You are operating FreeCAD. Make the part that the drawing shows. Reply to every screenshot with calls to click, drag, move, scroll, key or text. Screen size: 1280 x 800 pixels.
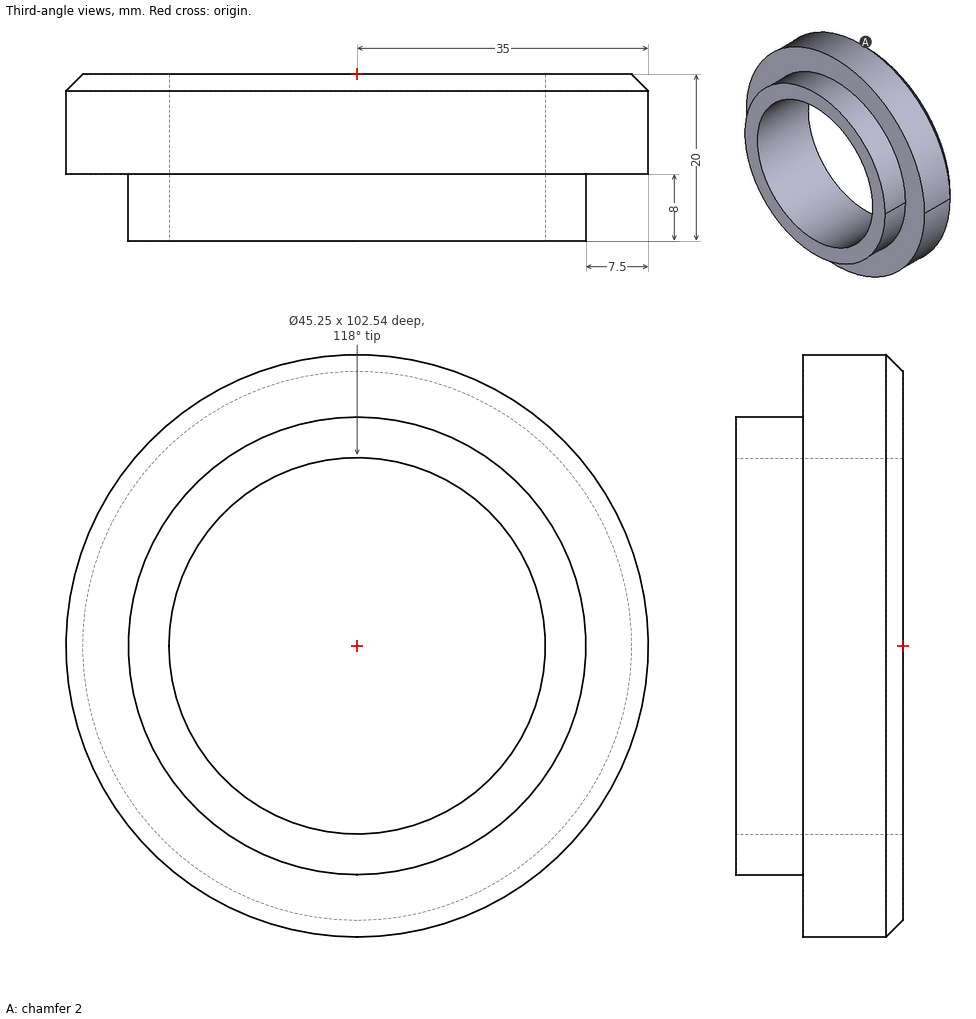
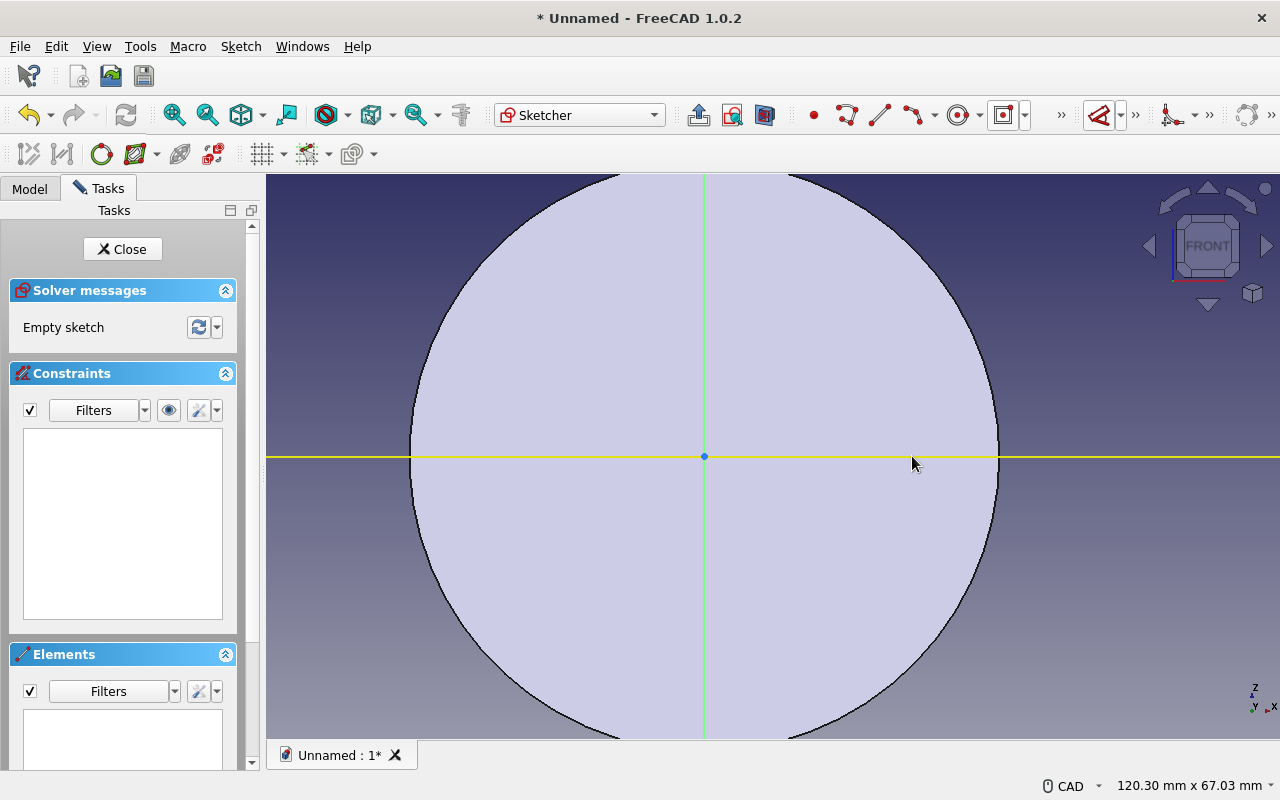
click(958, 116)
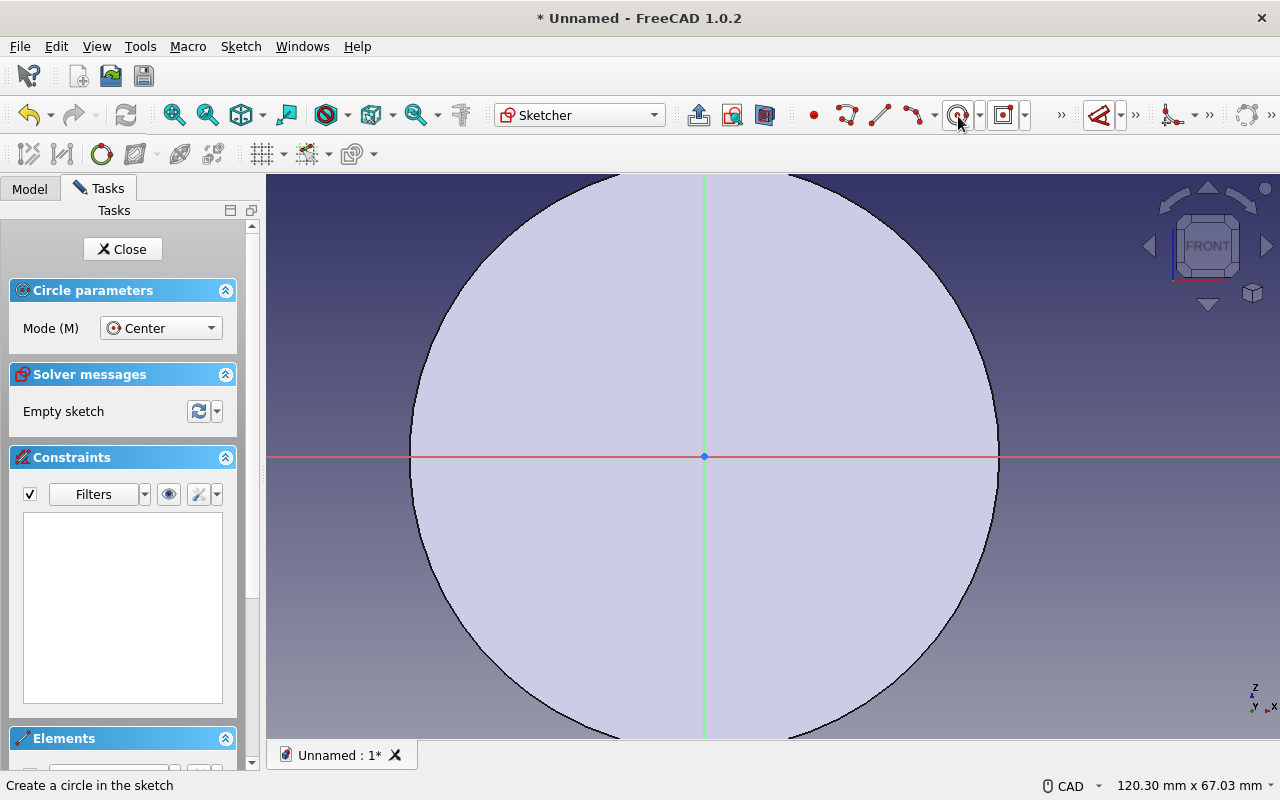
click(704, 456)
click(839, 322)
key(Escape)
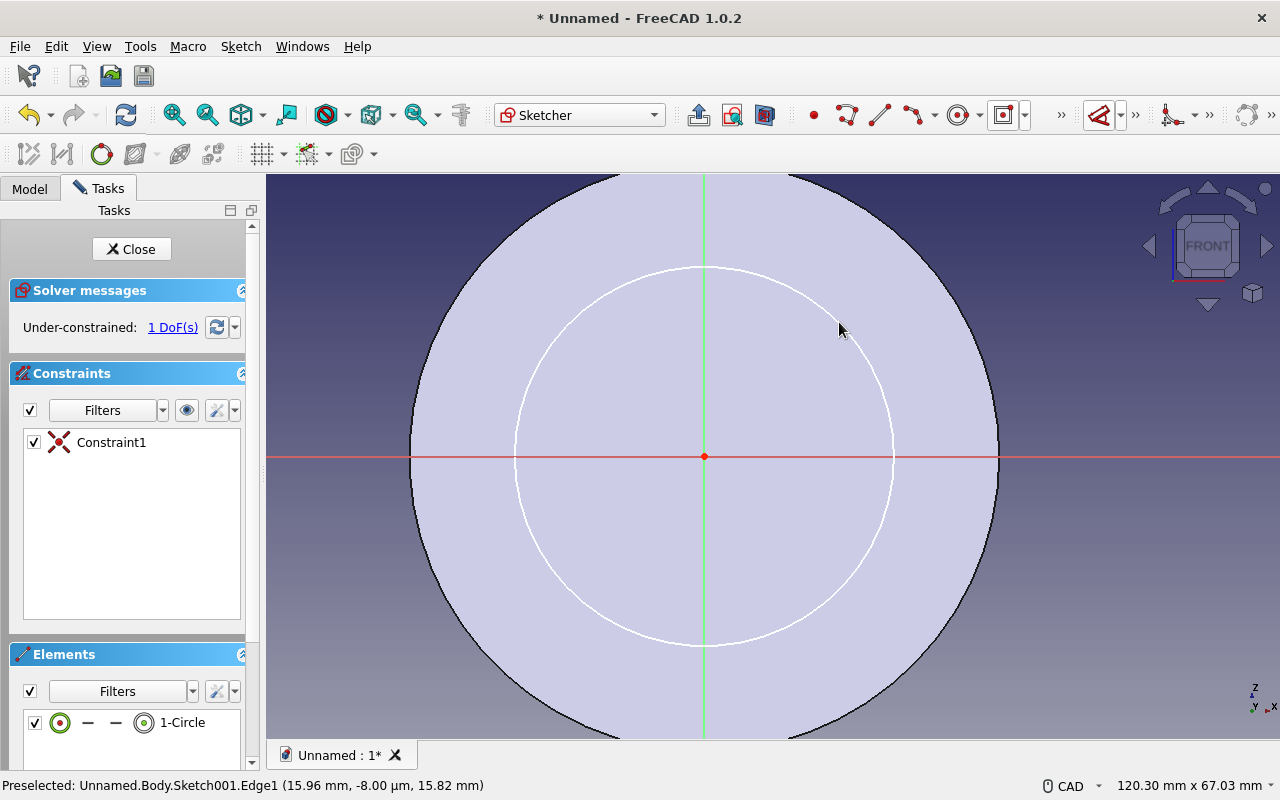
click(838, 322)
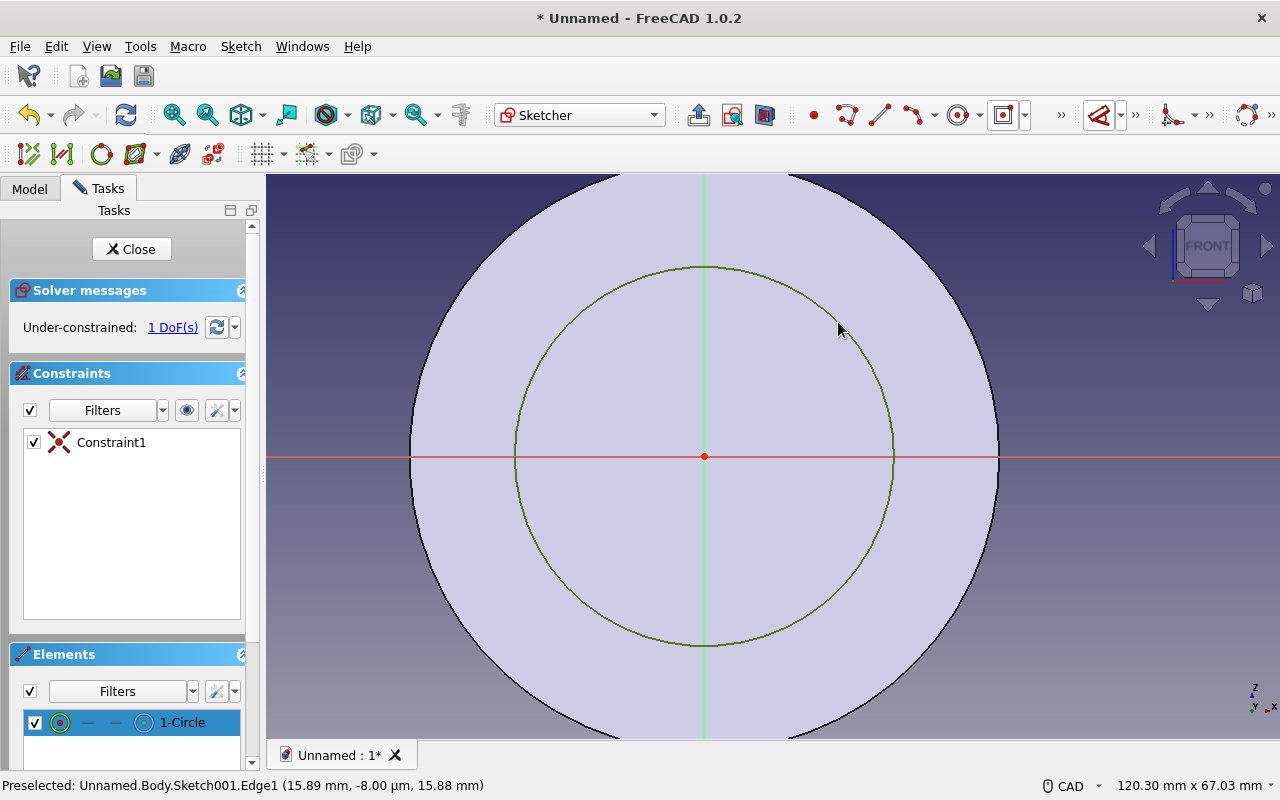
click(1120, 116)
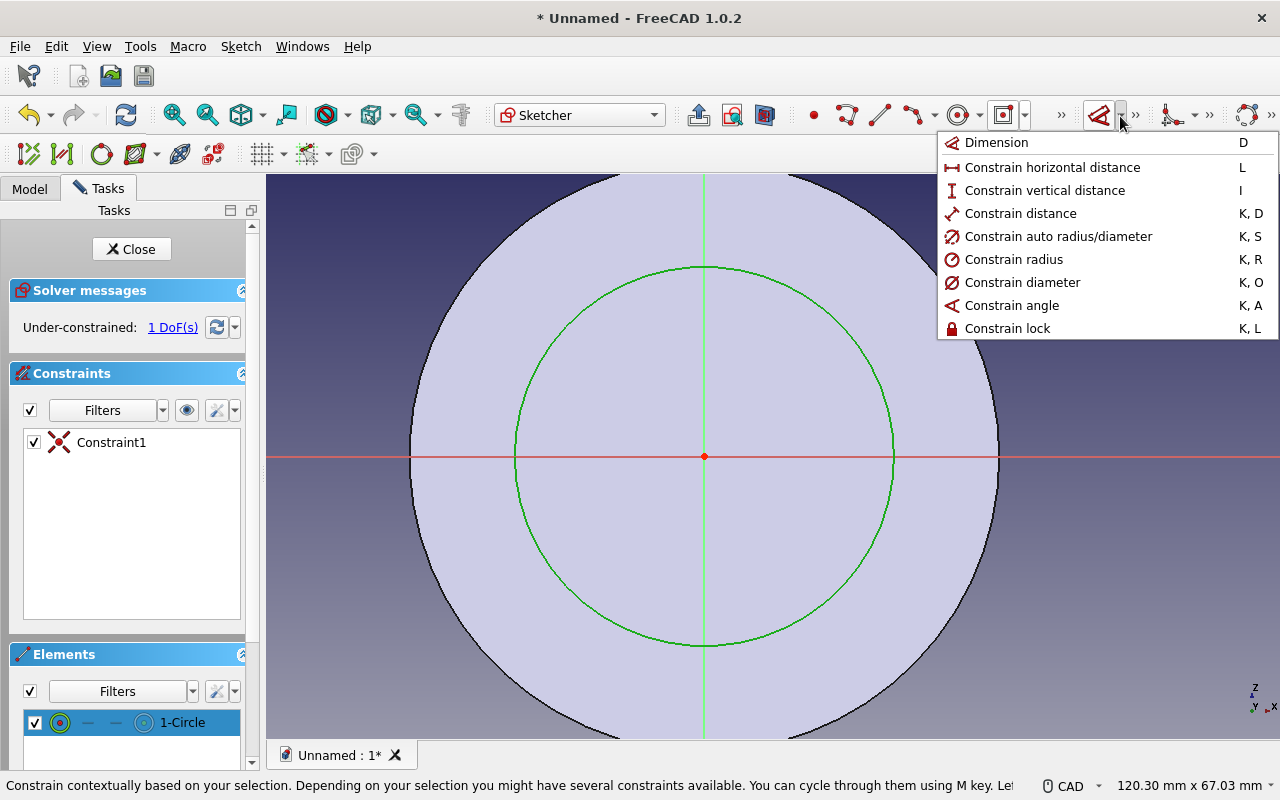
click(1108, 282)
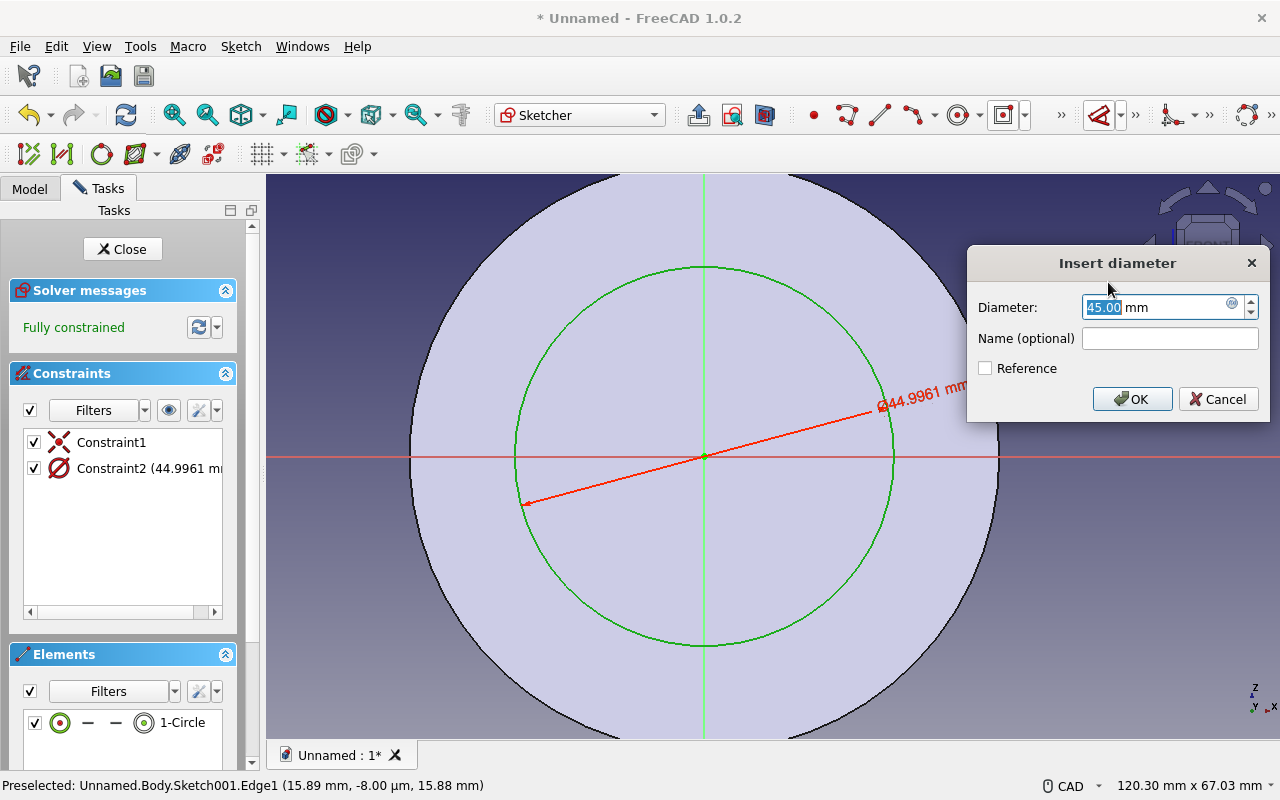
text(45.25)
key(Return)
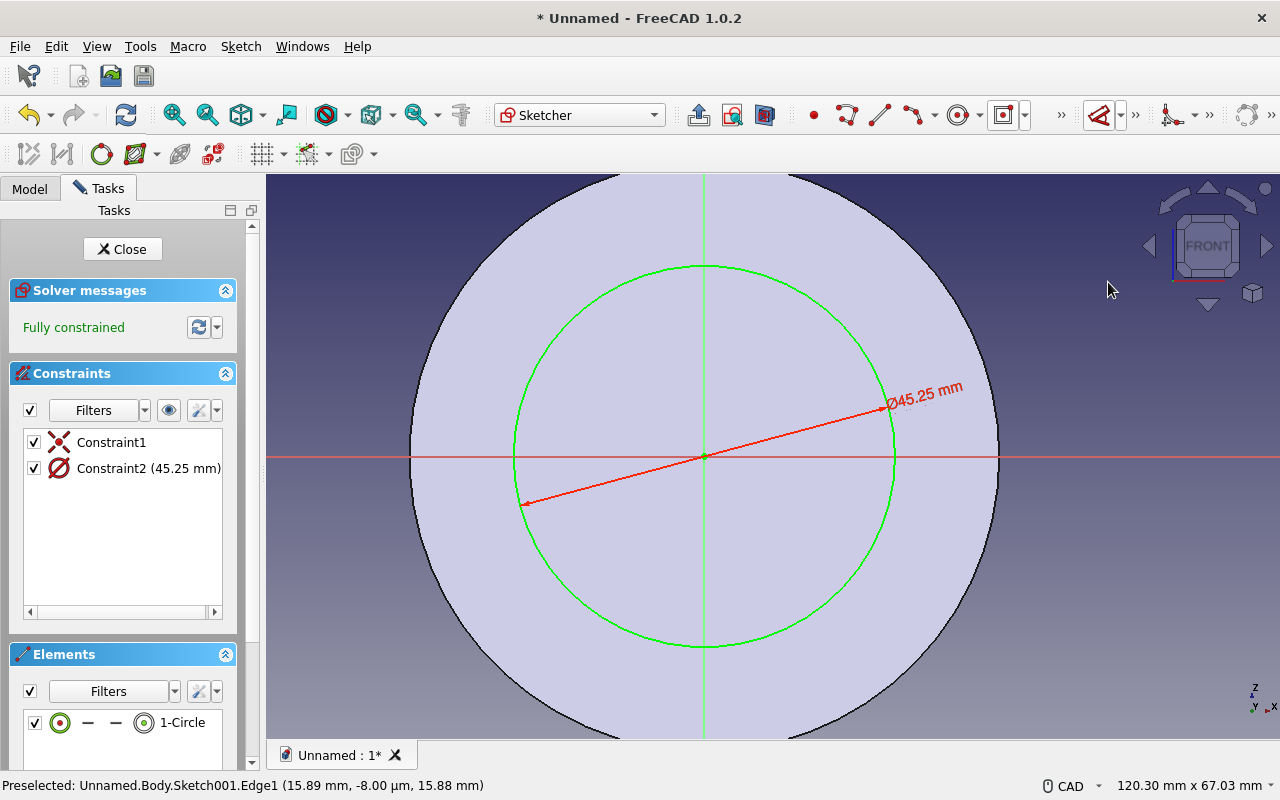
click(123, 249)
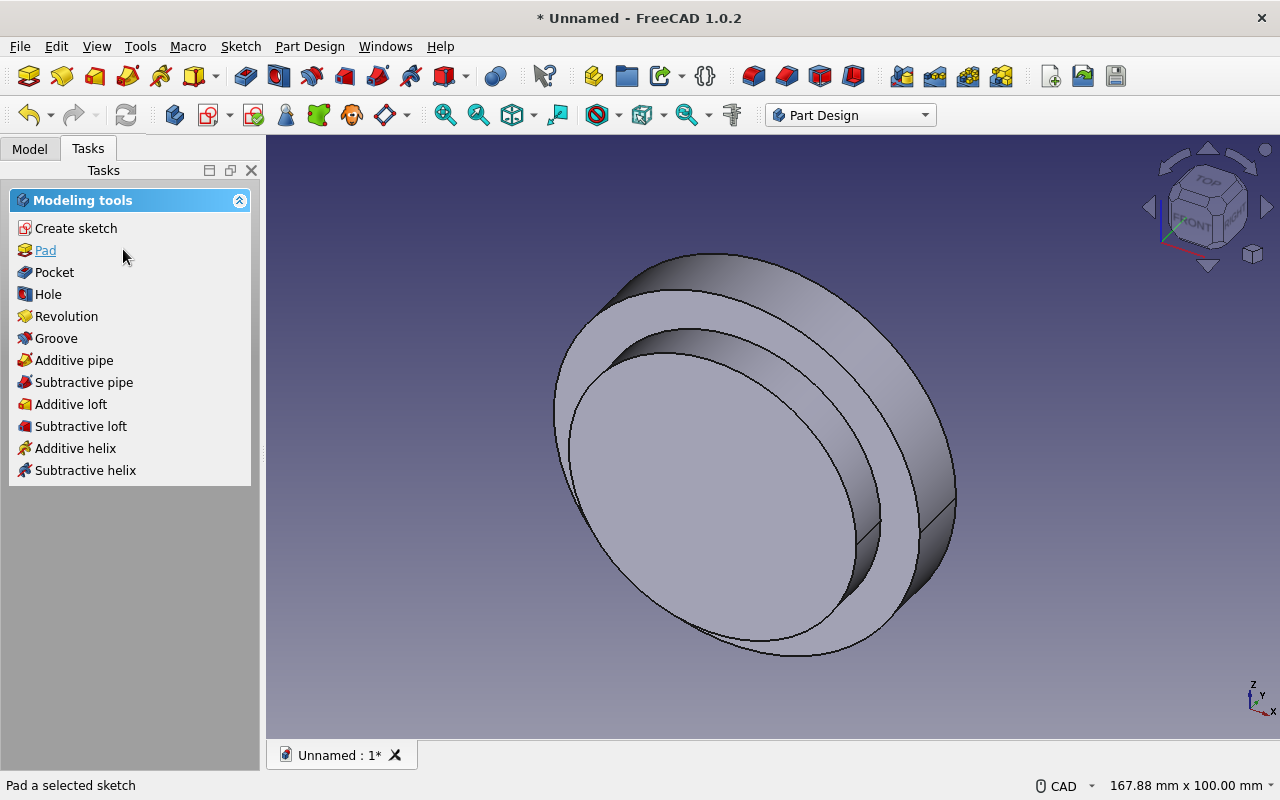
click(279, 76)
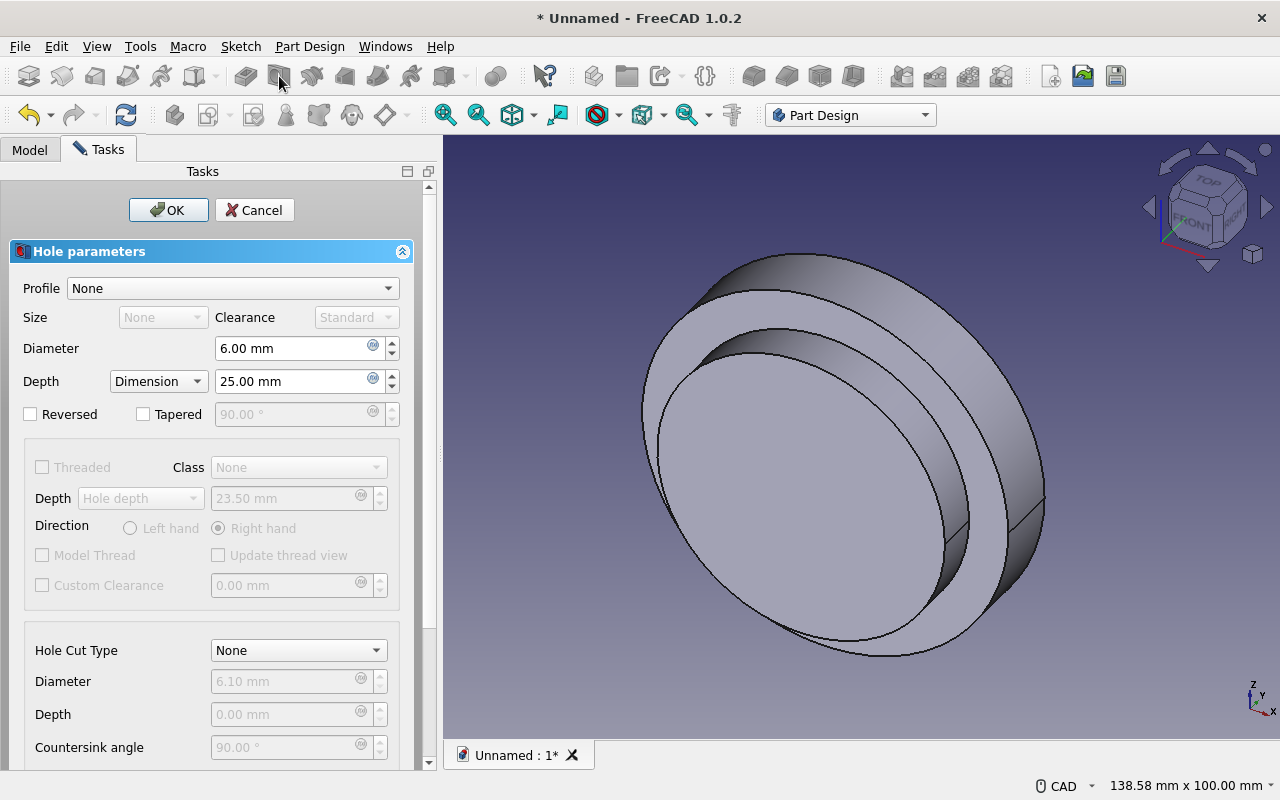
triple_click(300, 348)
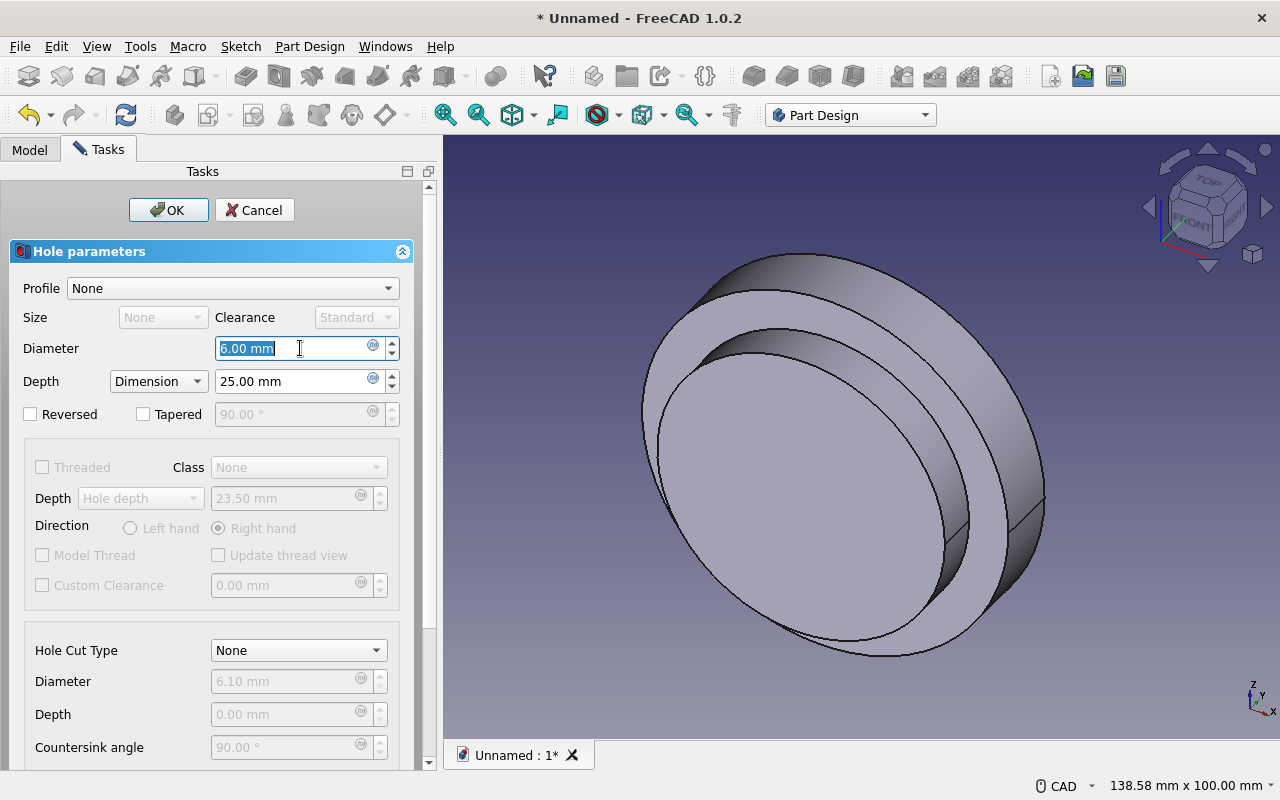
text(45.25)
key(Tab)